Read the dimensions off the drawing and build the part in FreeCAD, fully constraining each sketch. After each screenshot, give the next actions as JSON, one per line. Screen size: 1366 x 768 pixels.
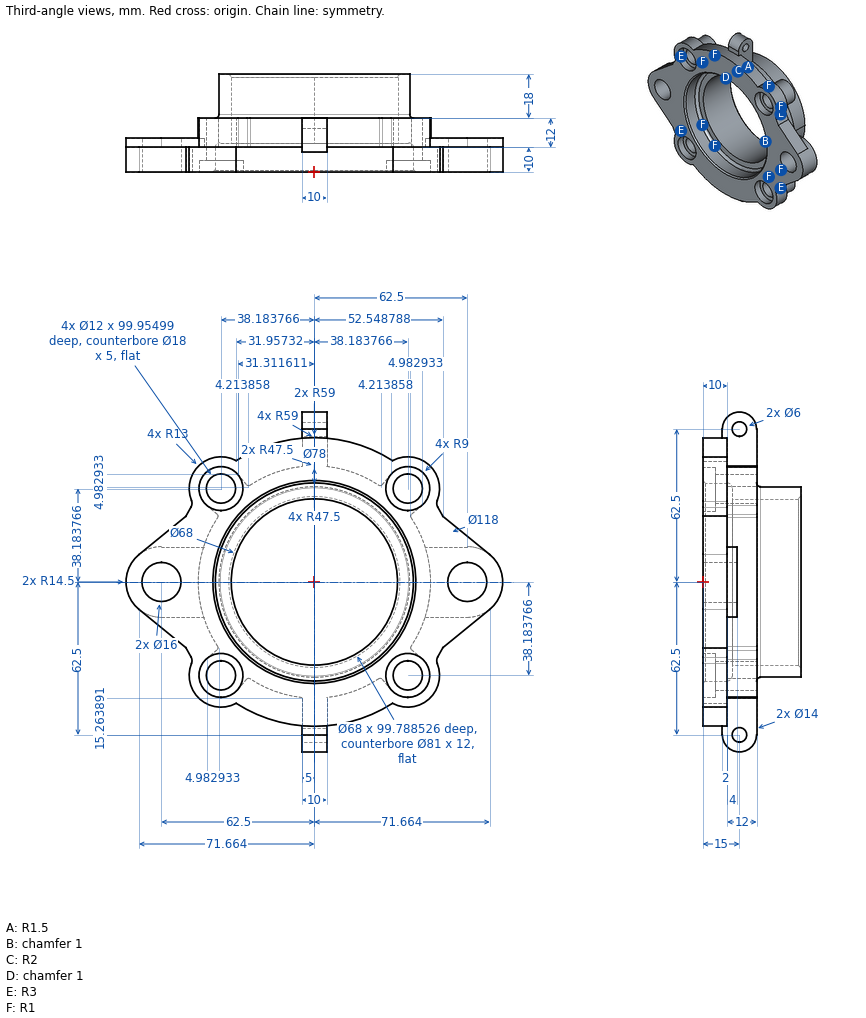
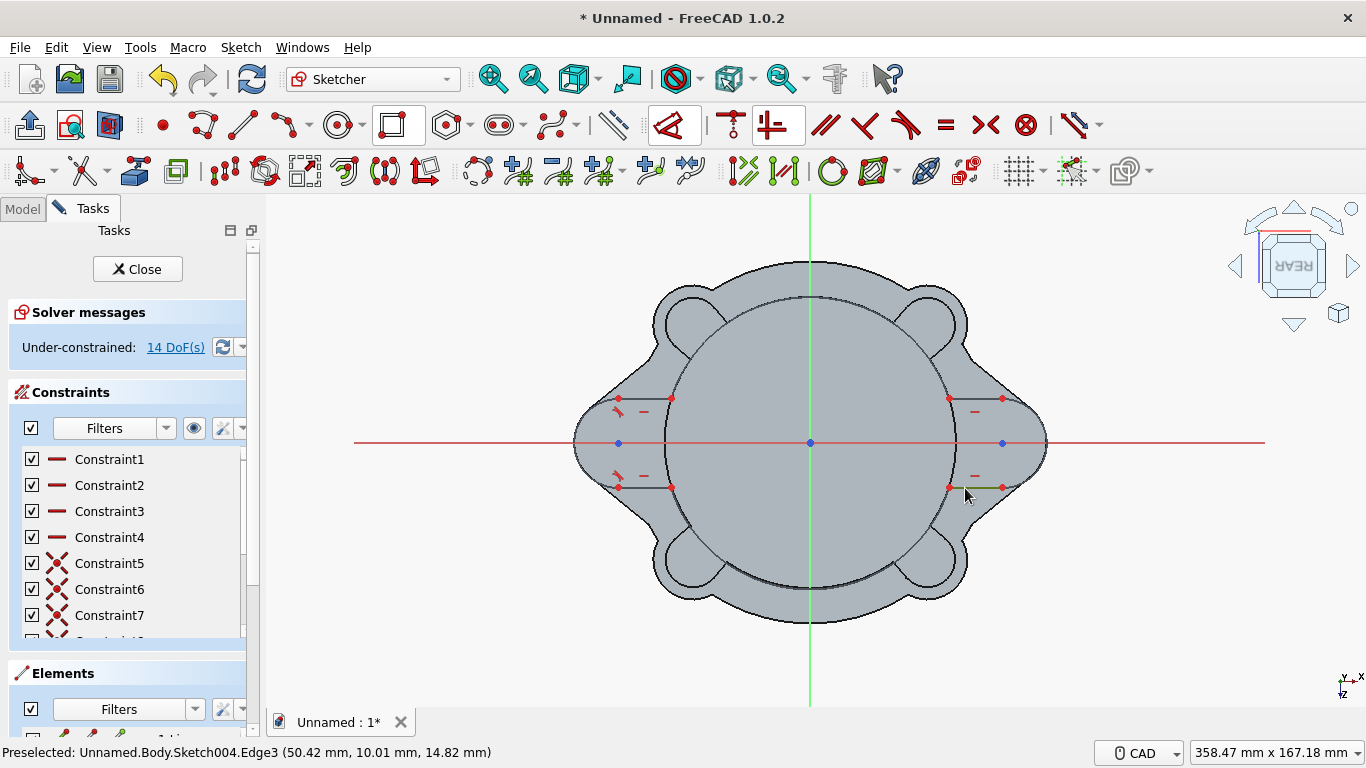
{"action": "left_click", "coordinate": [1038, 470]}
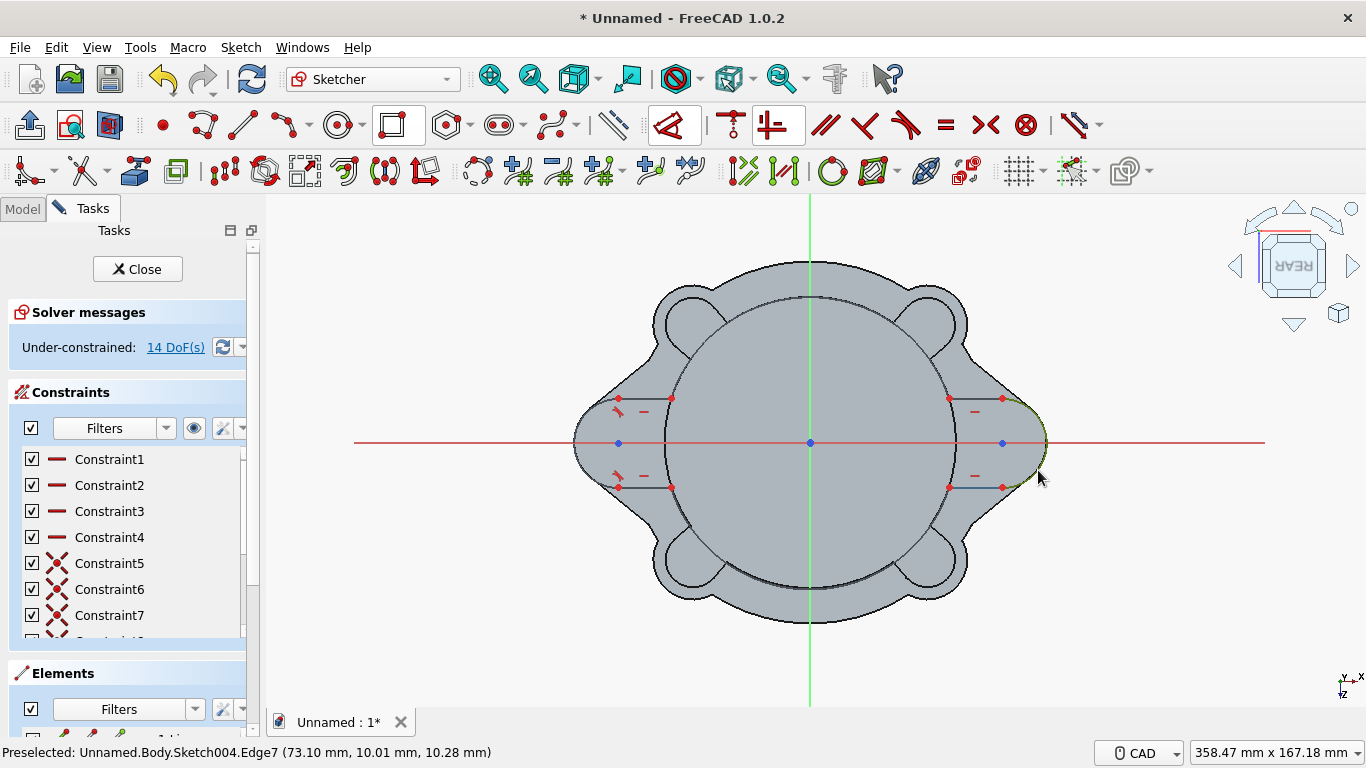
{"action": "left_click", "coordinate": [906, 126]}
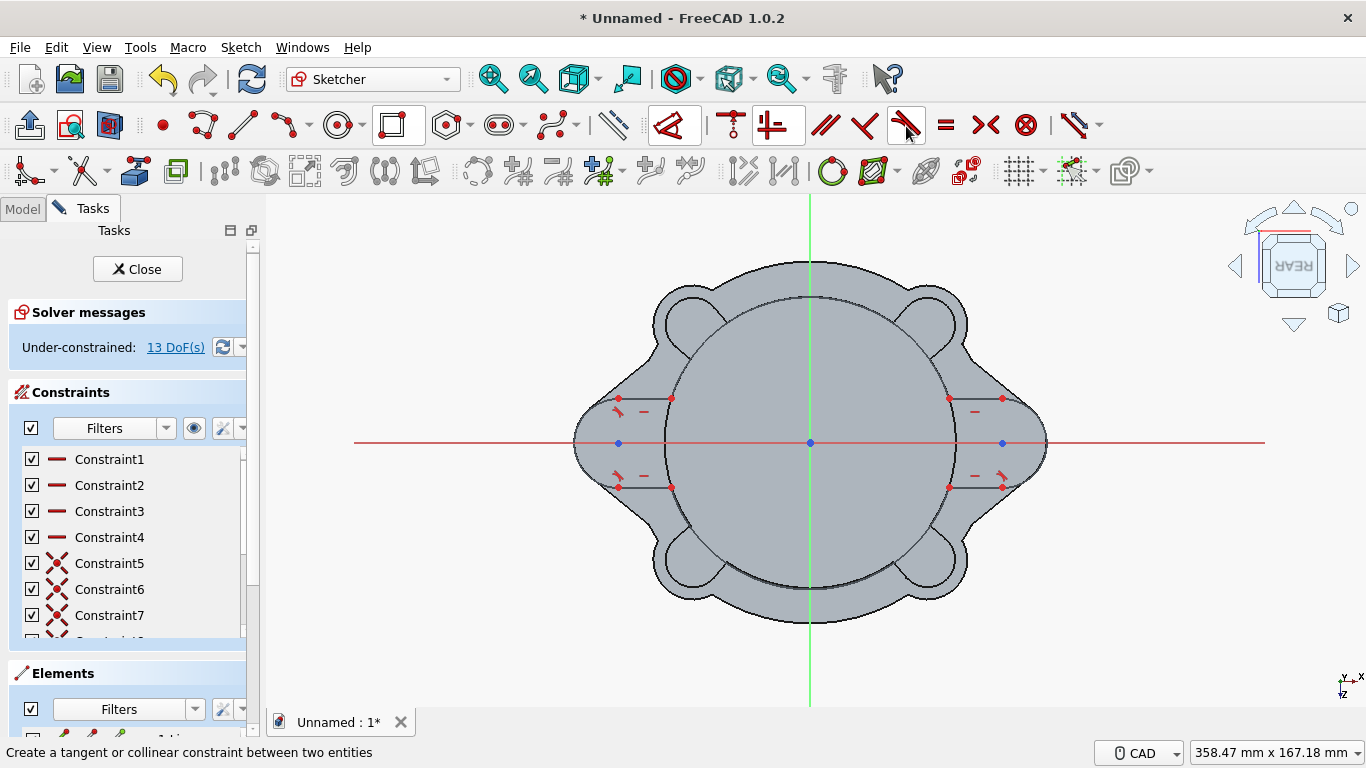
{"action": "left_click", "coordinate": [986, 399]}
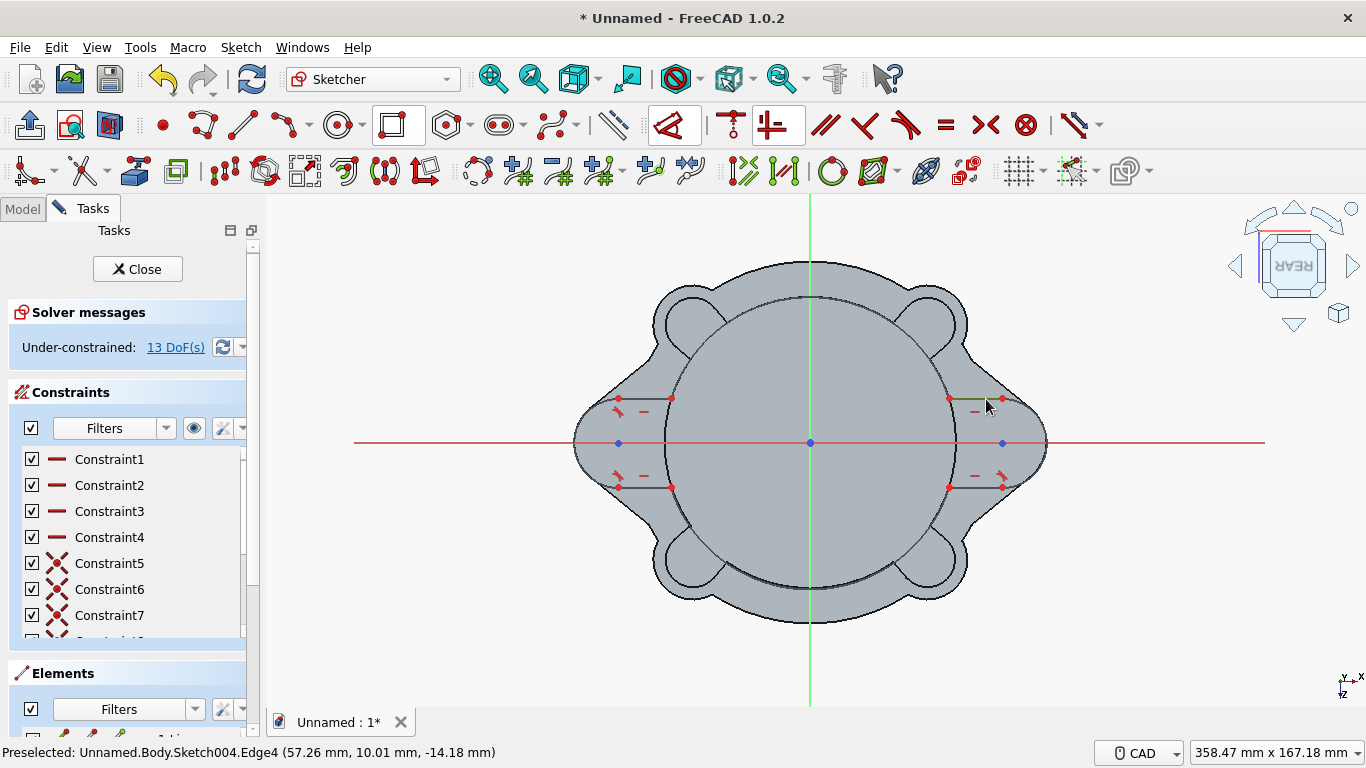
{"action": "left_click", "coordinate": [1038, 470]}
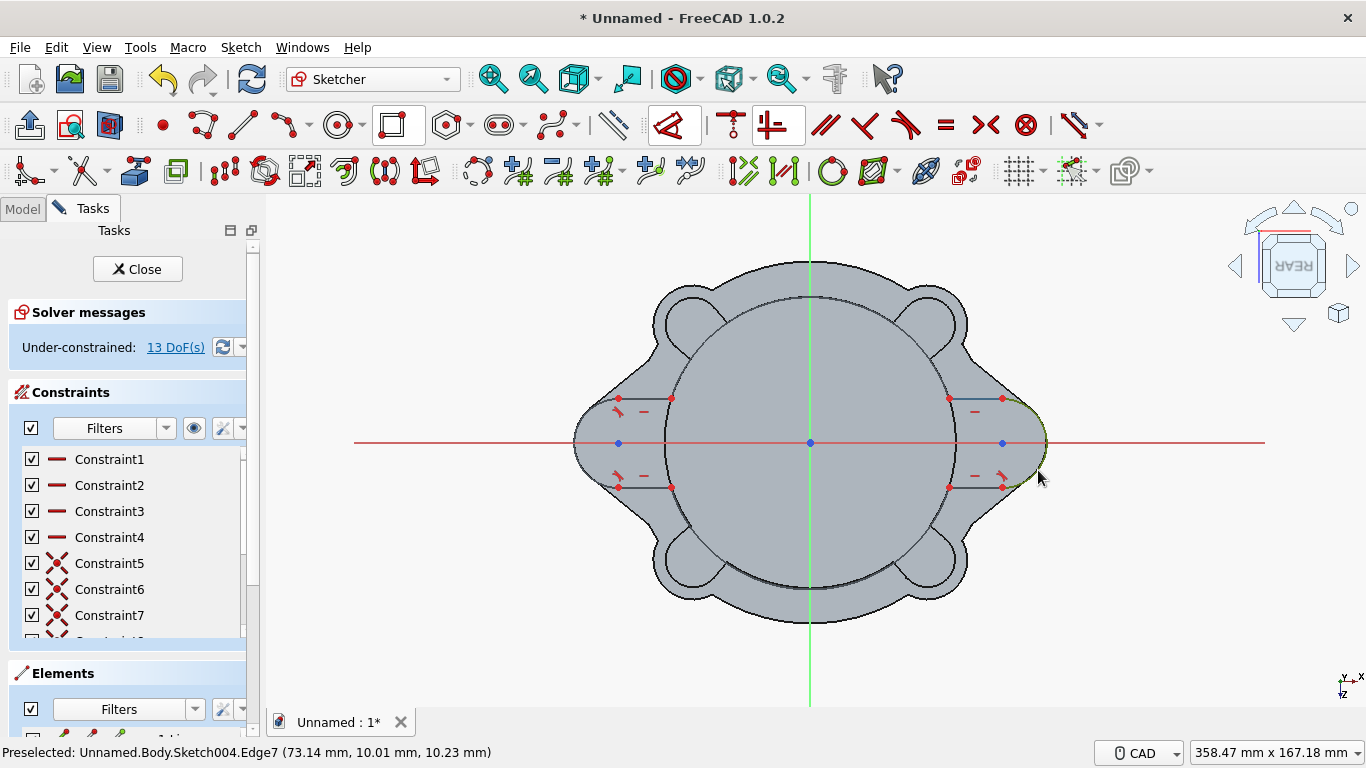
{"action": "left_click", "coordinate": [906, 126]}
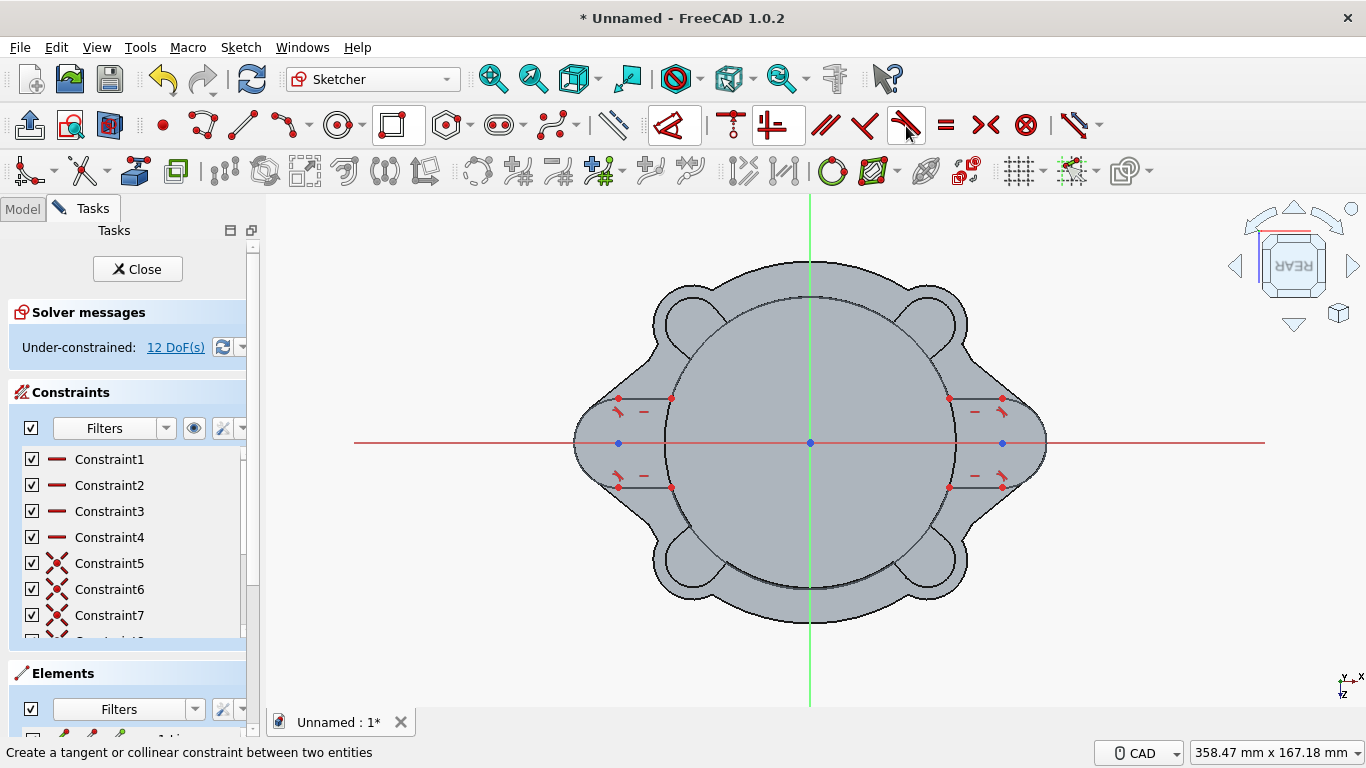
{"action": "left_click", "coordinate": [739, 571]}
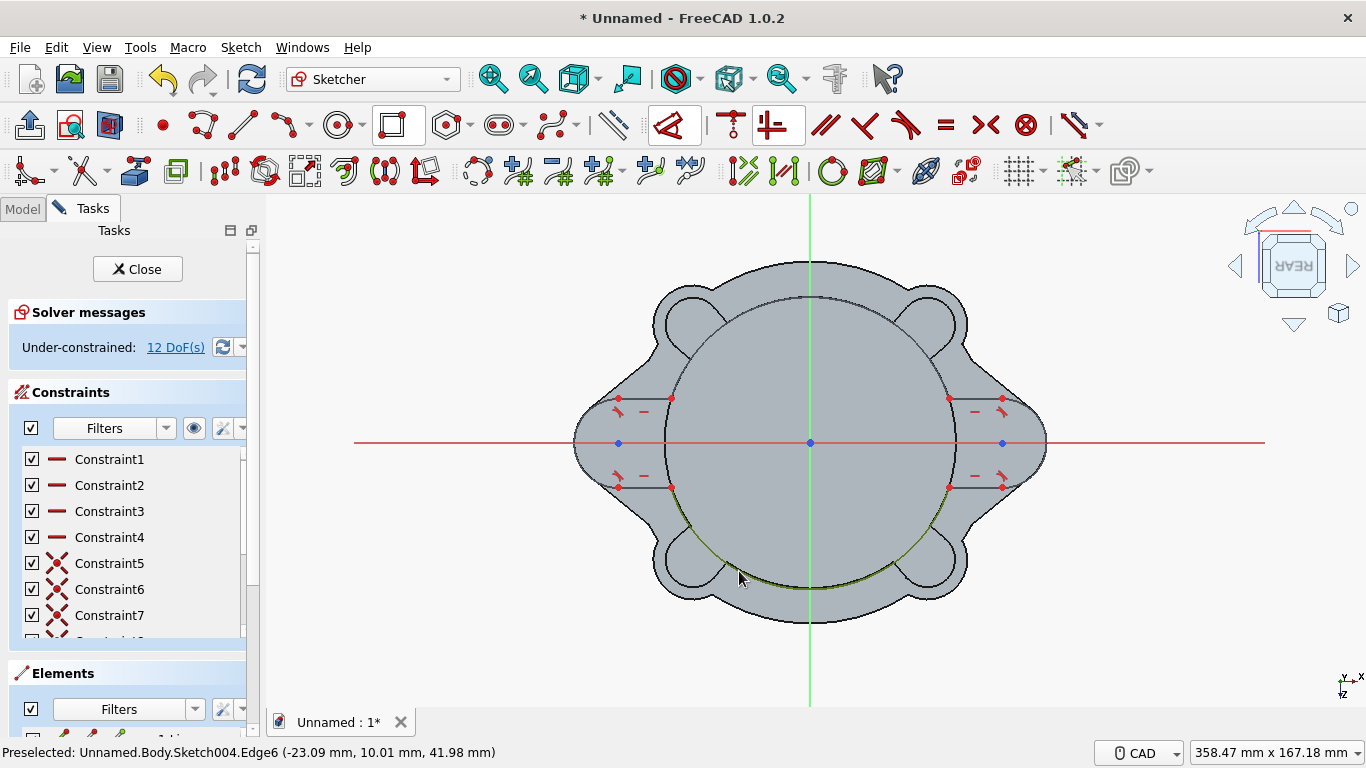
{"action": "left_click", "coordinate": [881, 315]}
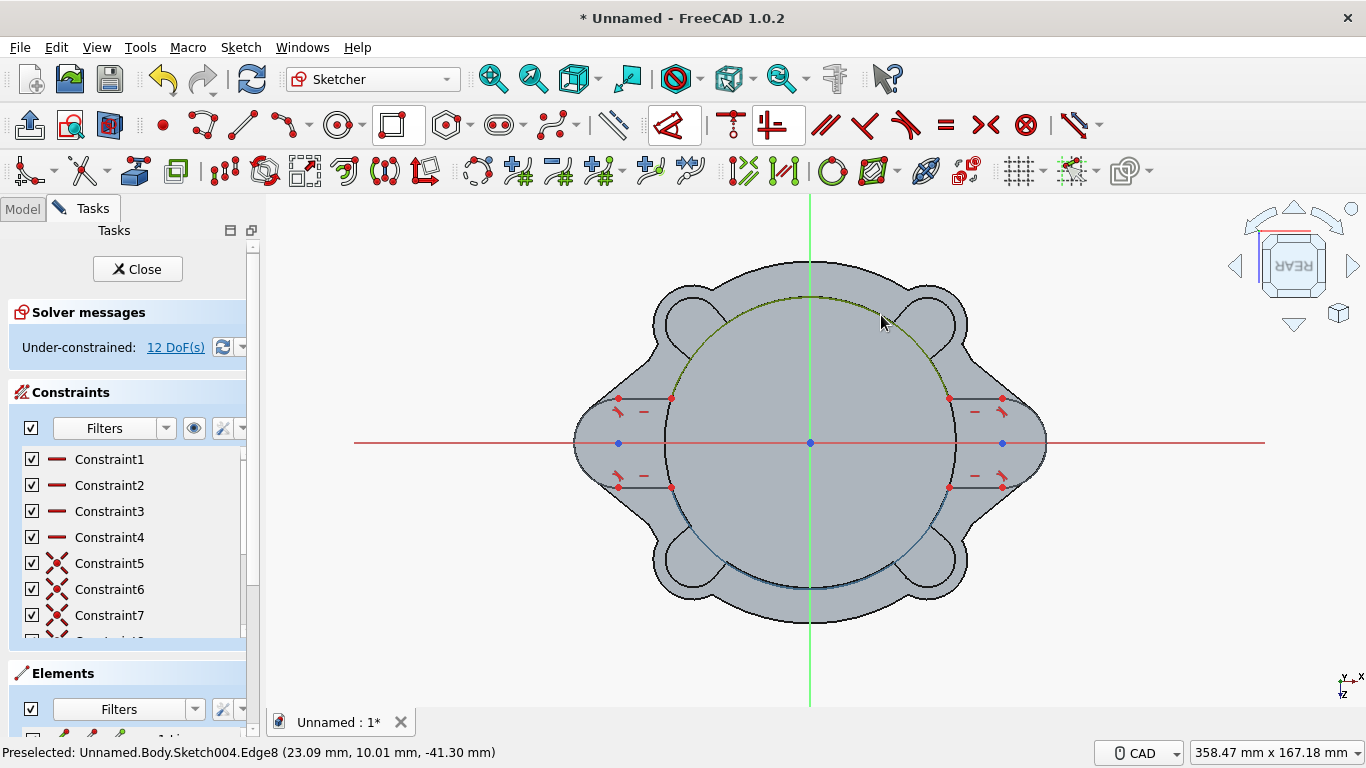
{"action": "left_click", "coordinate": [732, 126]}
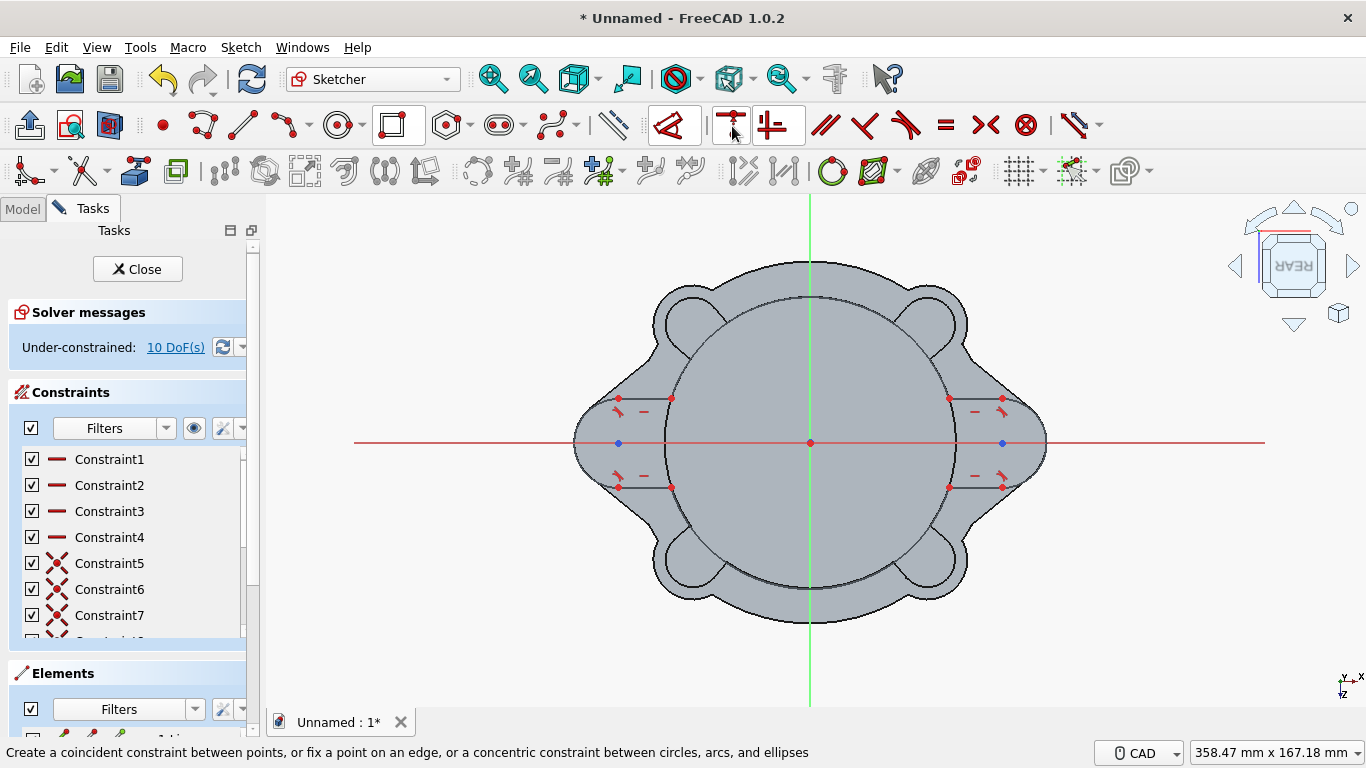
{"action": "left_click_drag", "start_coordinate": [800, 433], "coordinate": [820, 453]}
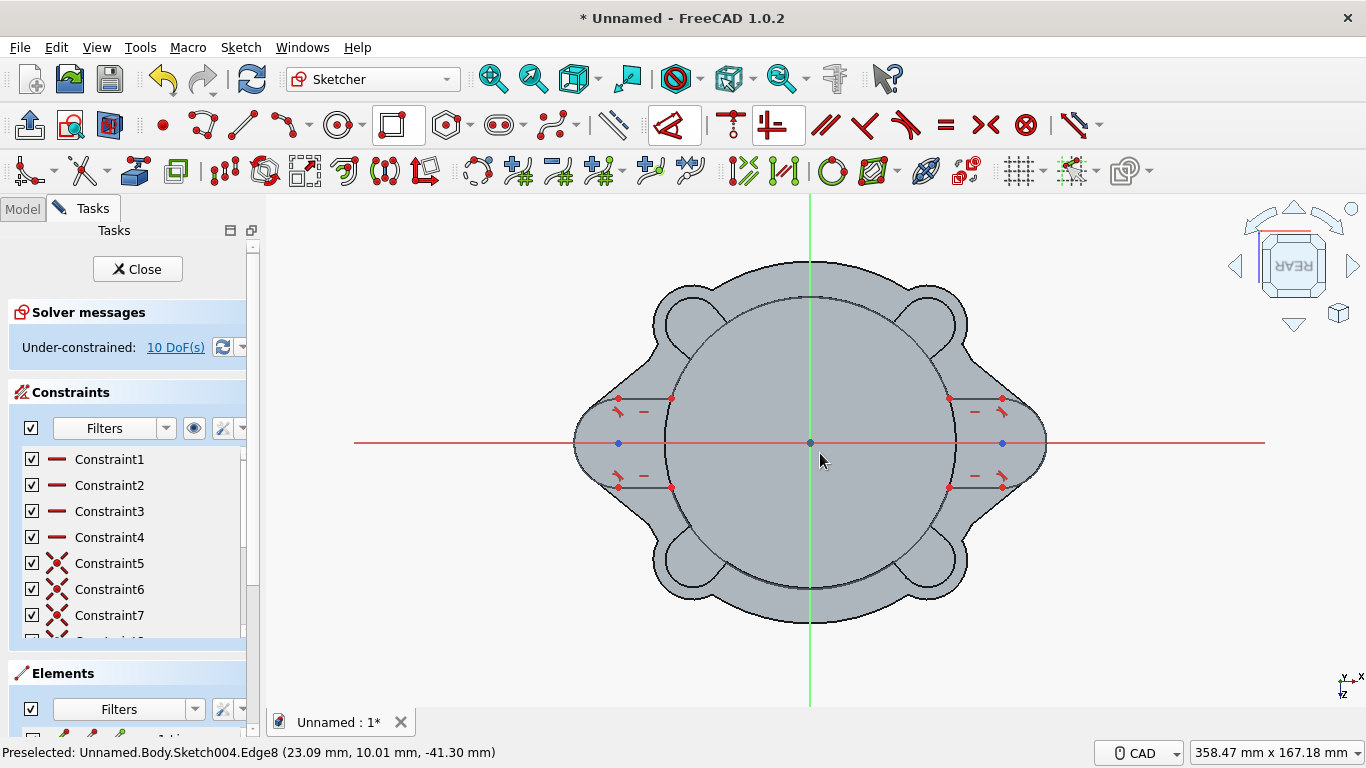
{"action": "left_click", "coordinate": [732, 126]}